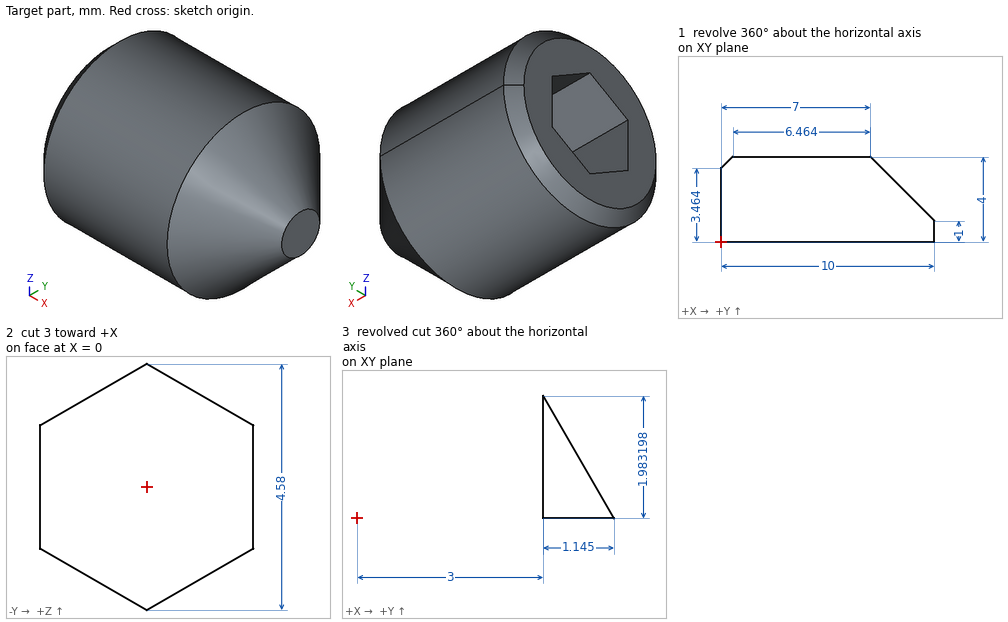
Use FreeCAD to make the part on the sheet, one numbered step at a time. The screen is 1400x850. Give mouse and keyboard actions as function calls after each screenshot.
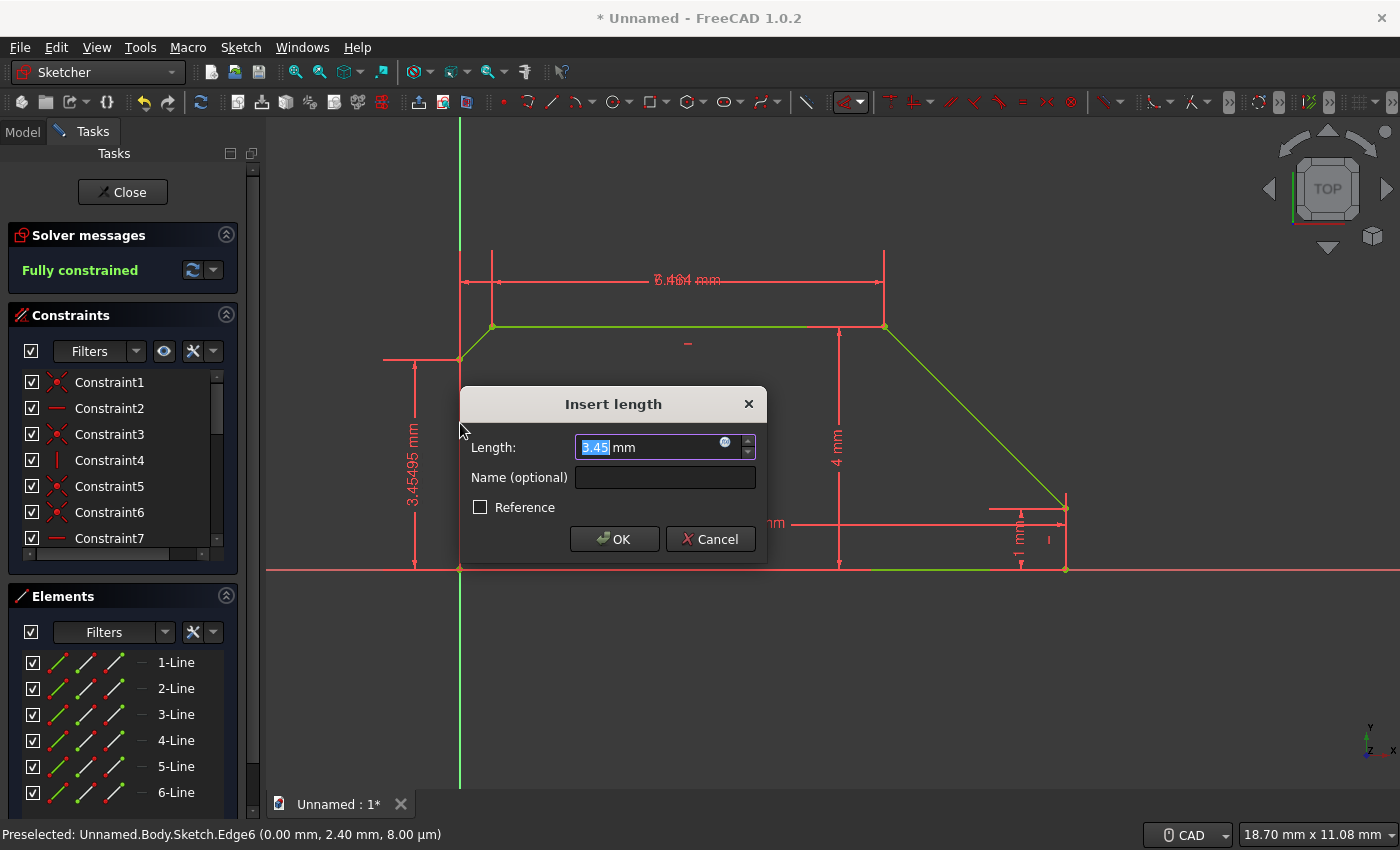
text(3.464)
key(Return)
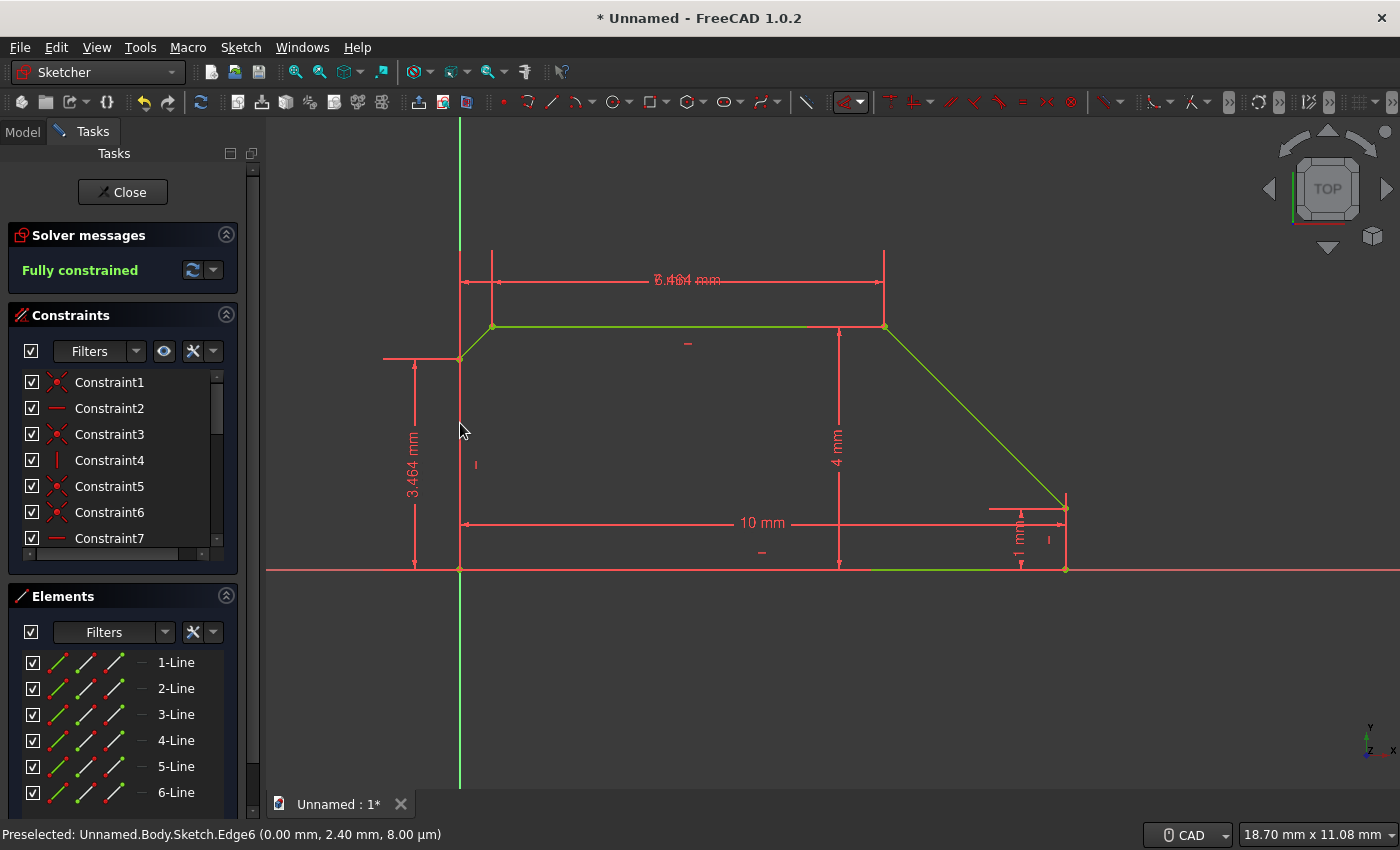
click(123, 192)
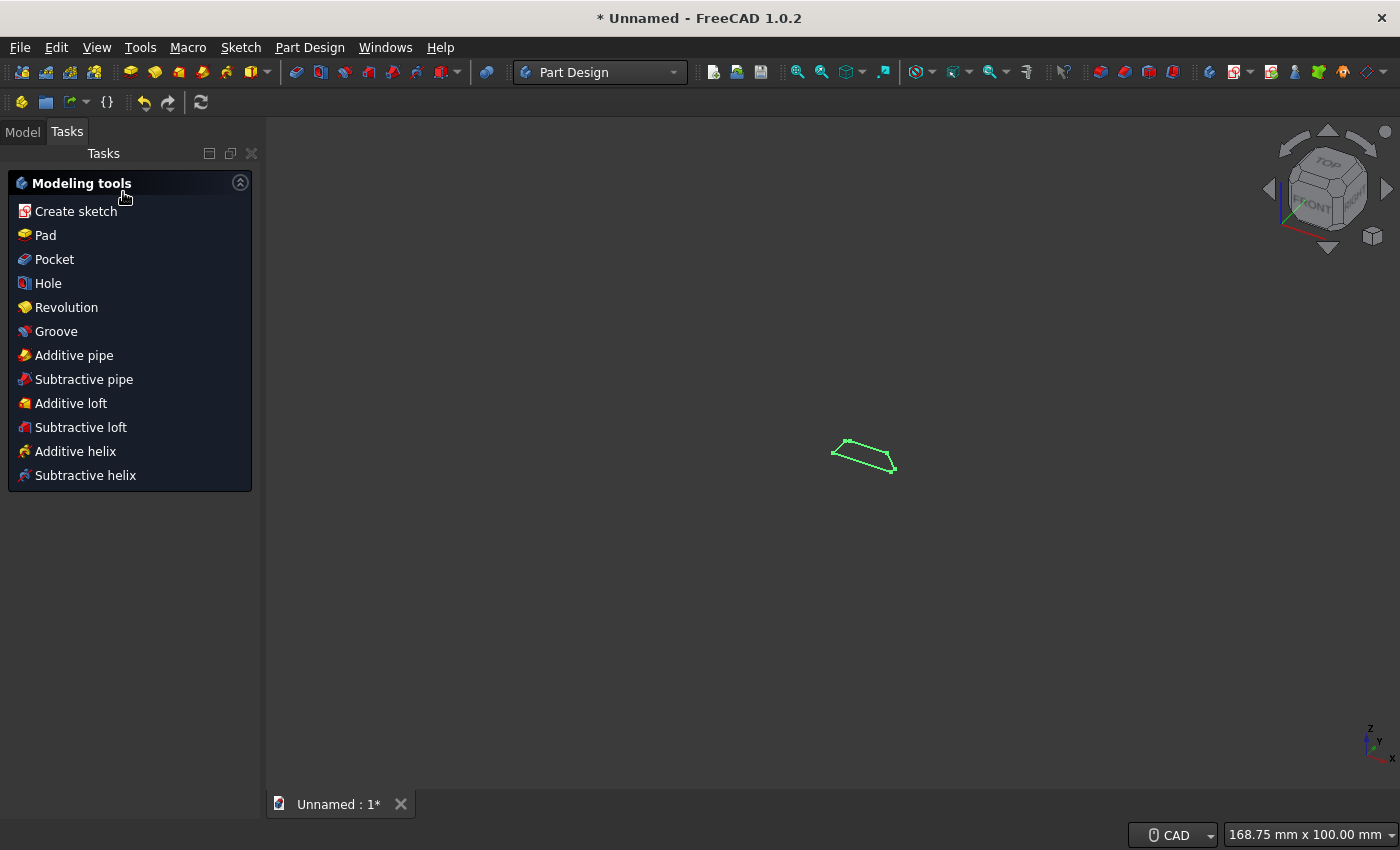
click(156, 72)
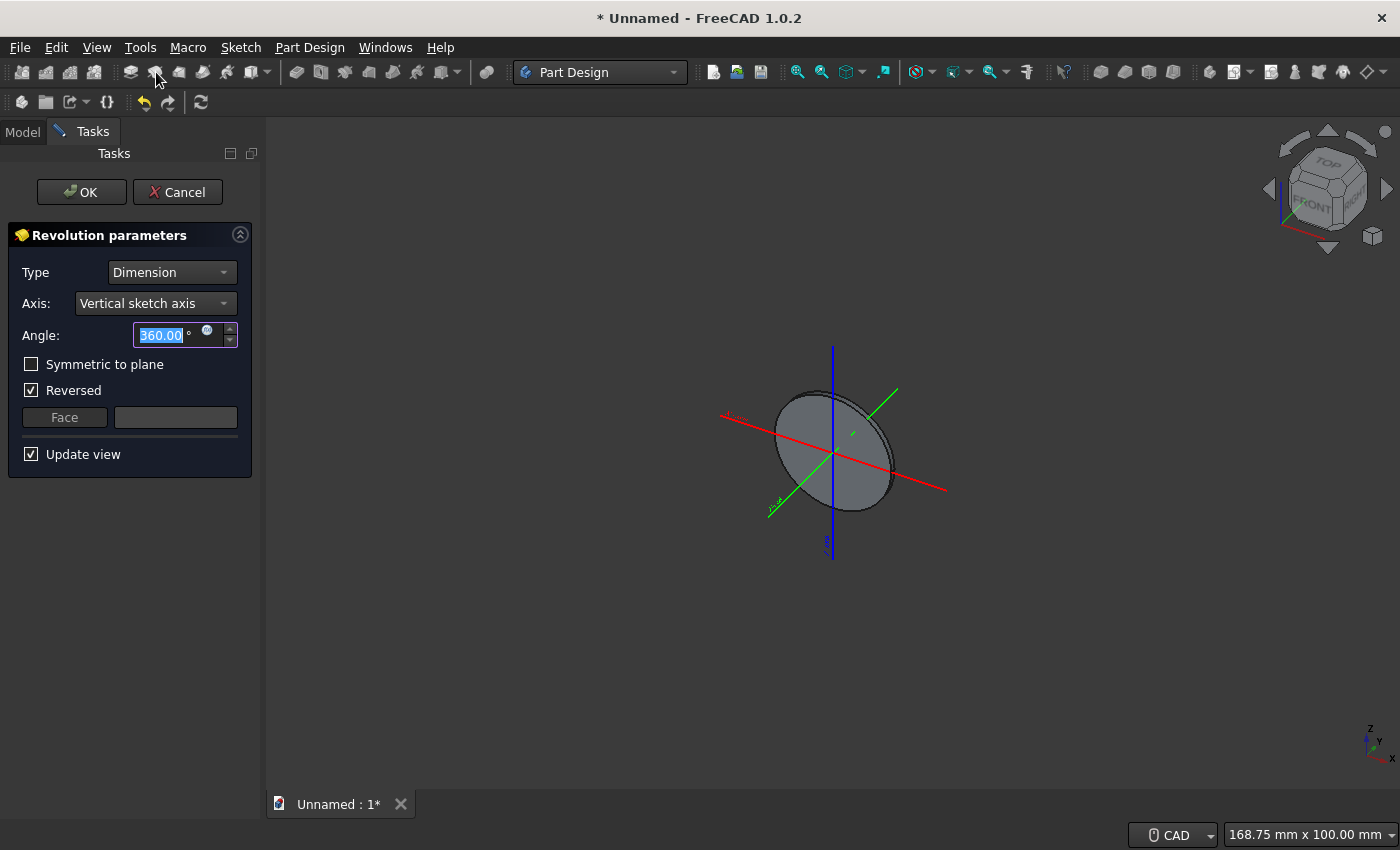
click(156, 304)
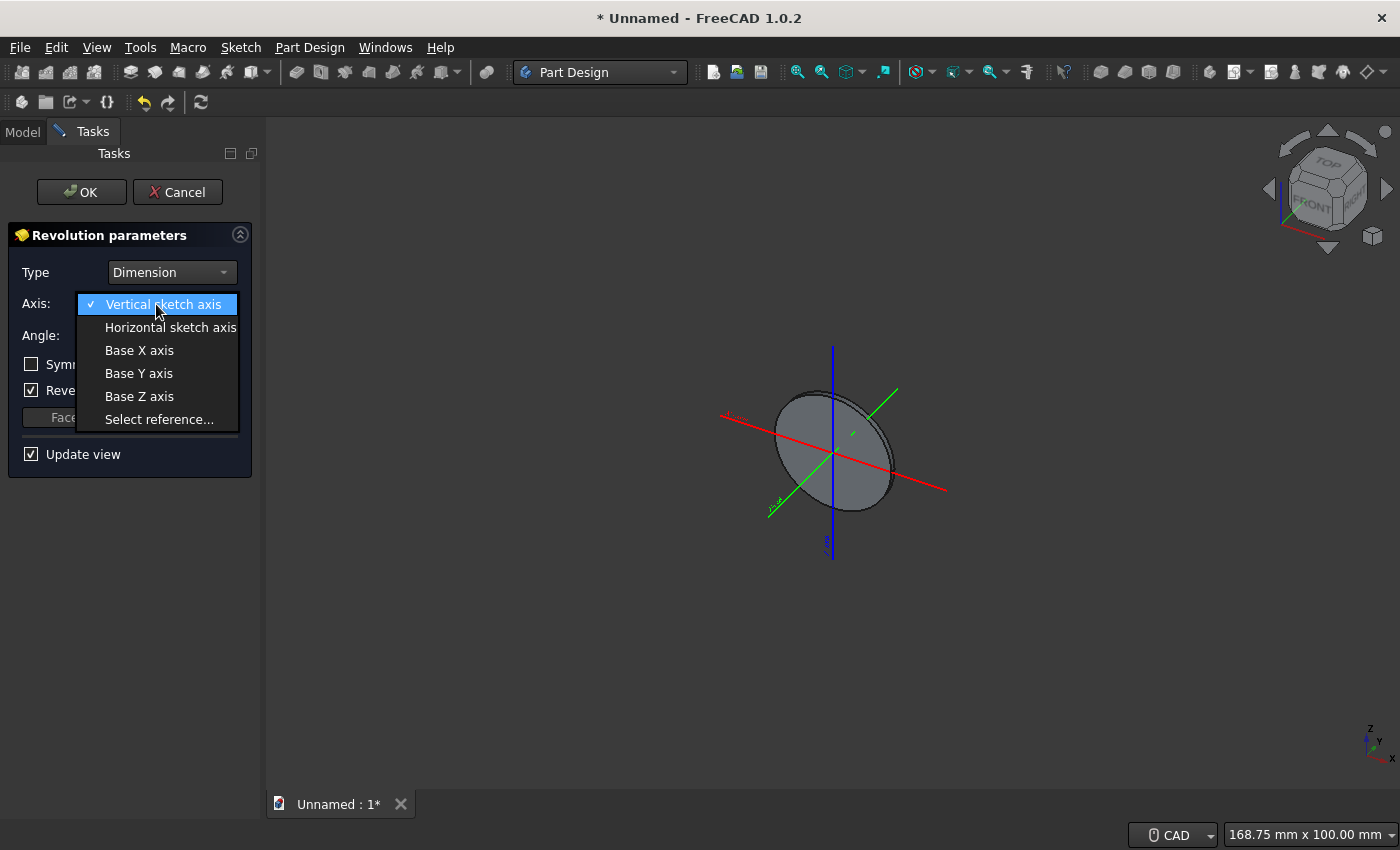
click(156, 328)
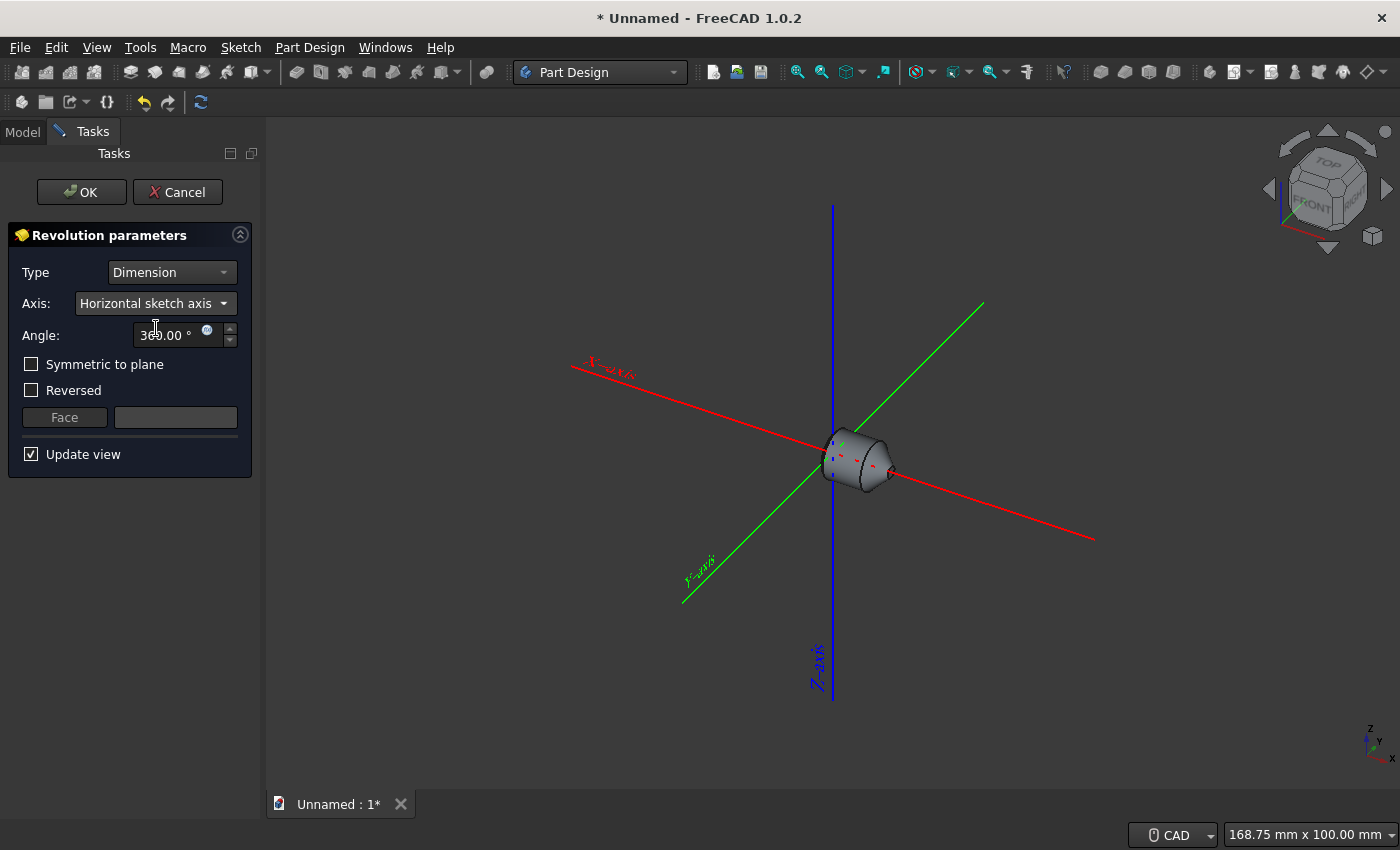
click(82, 192)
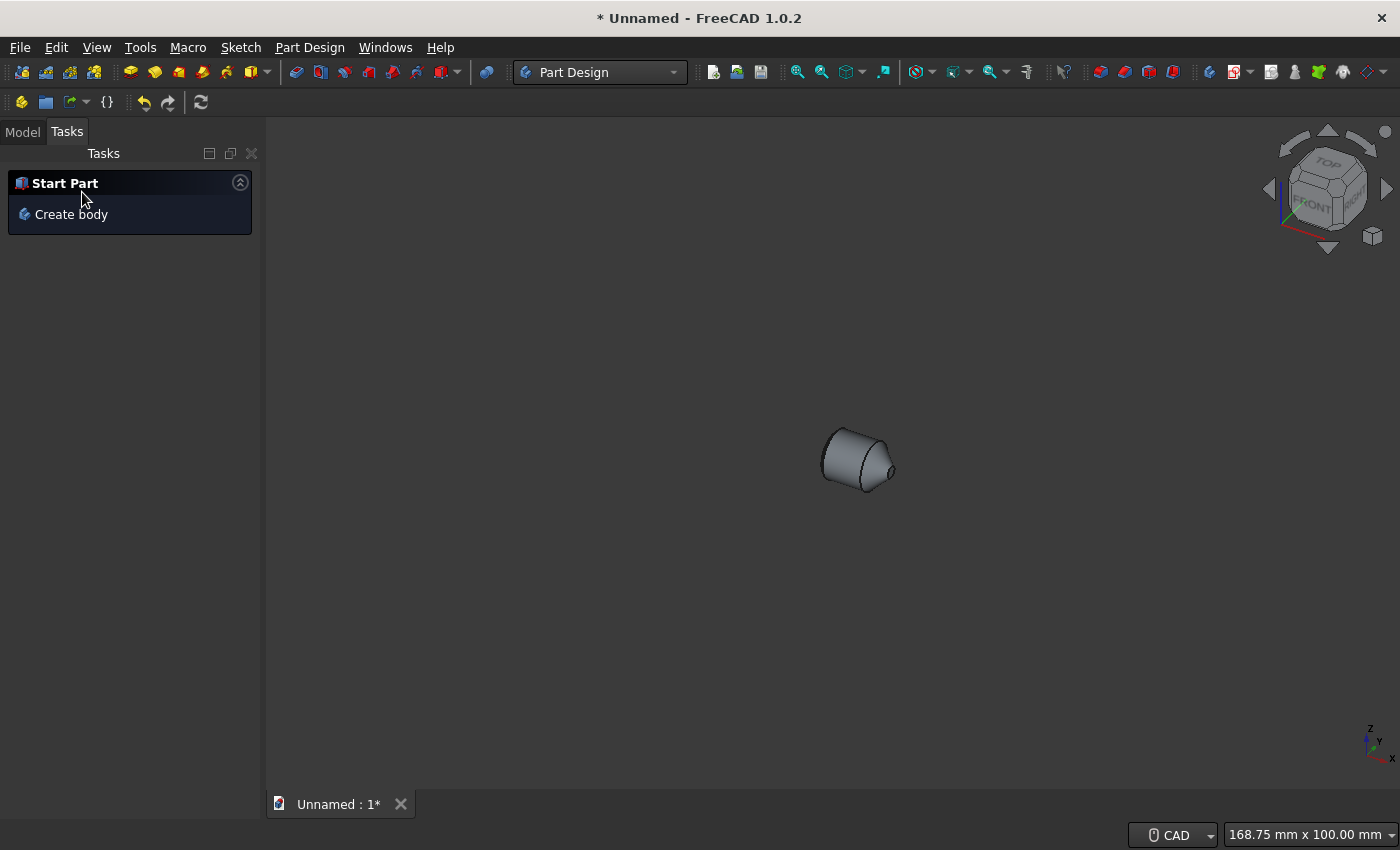
key(v)
key(f)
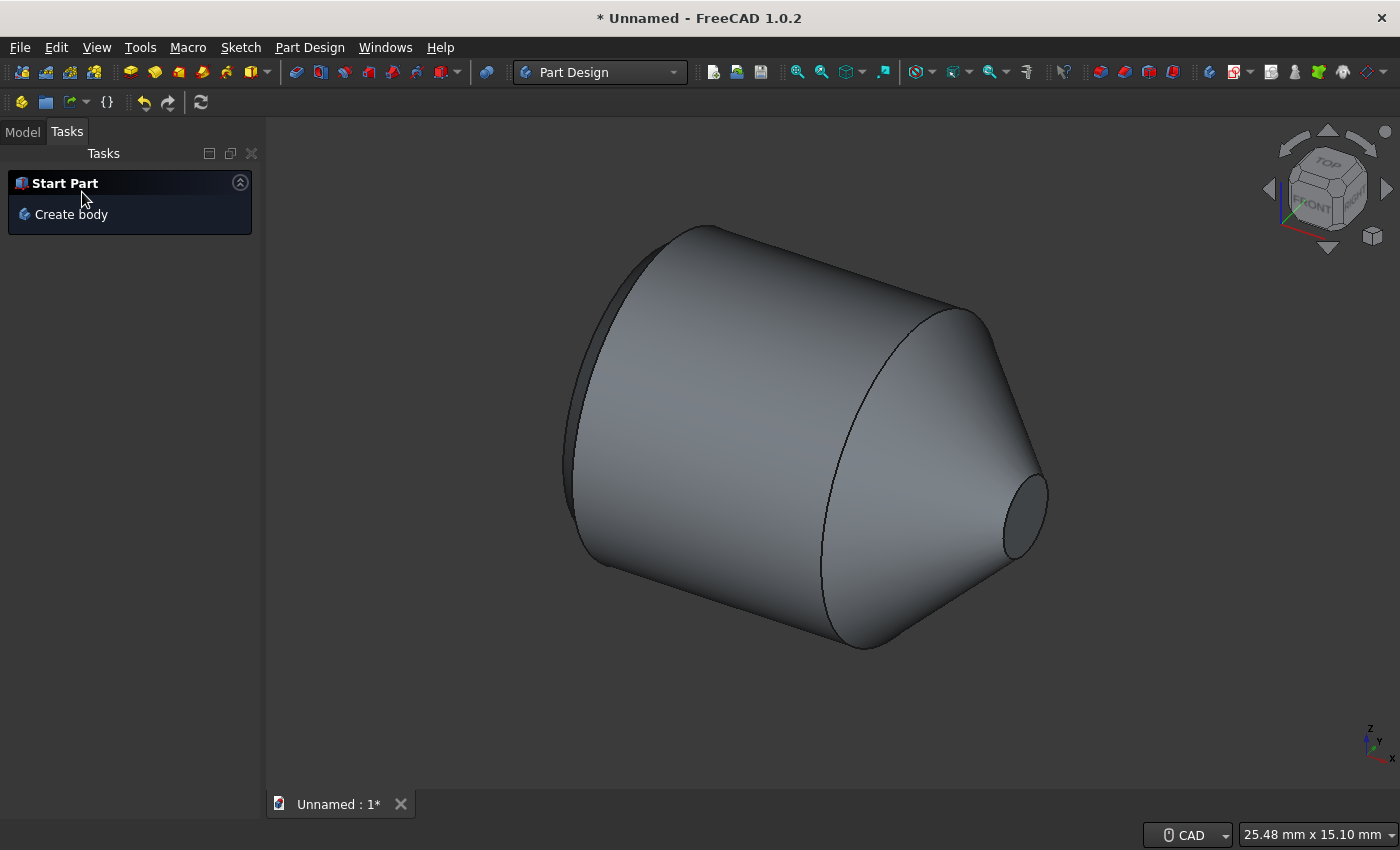
key(6)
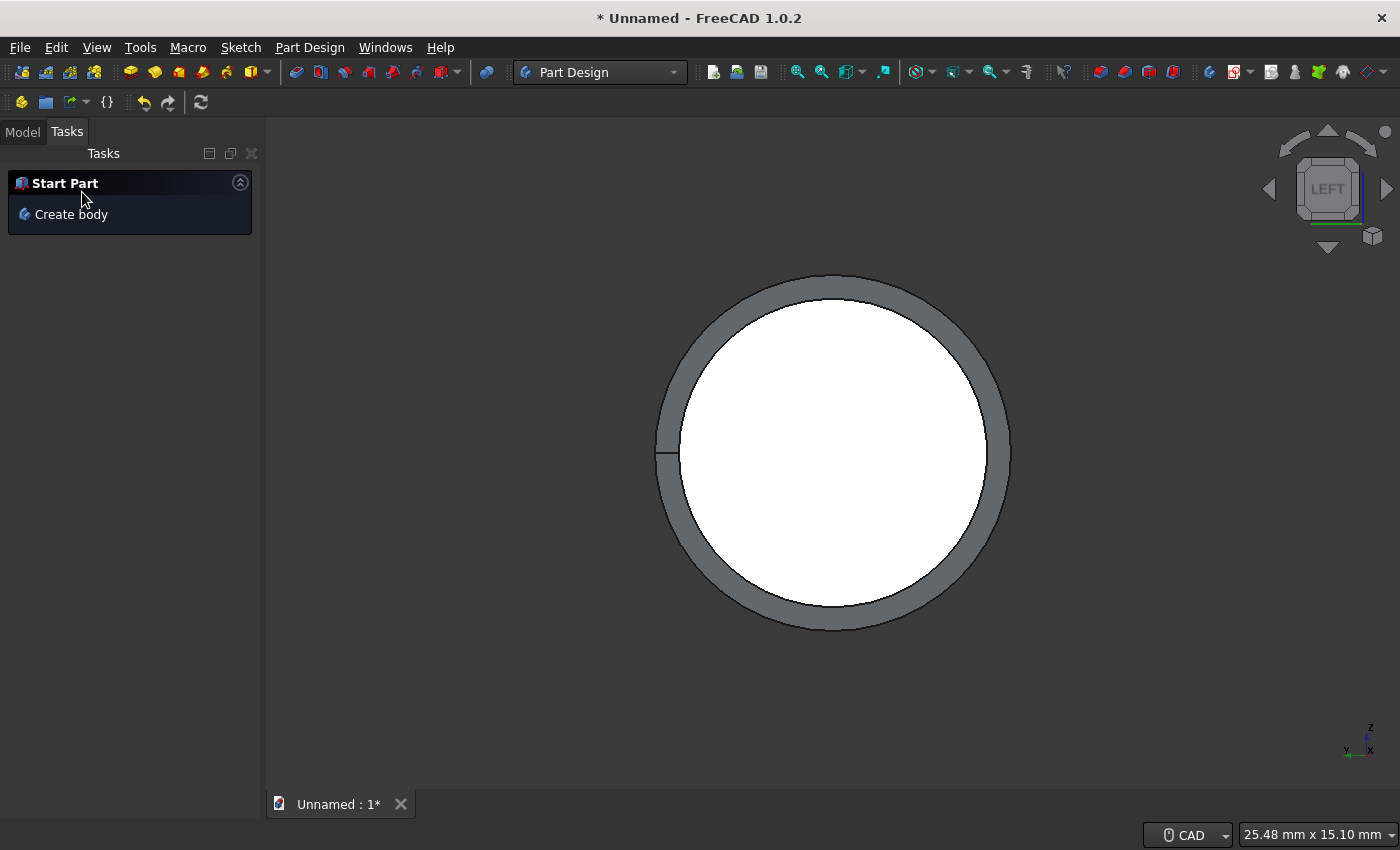
click(833, 452)